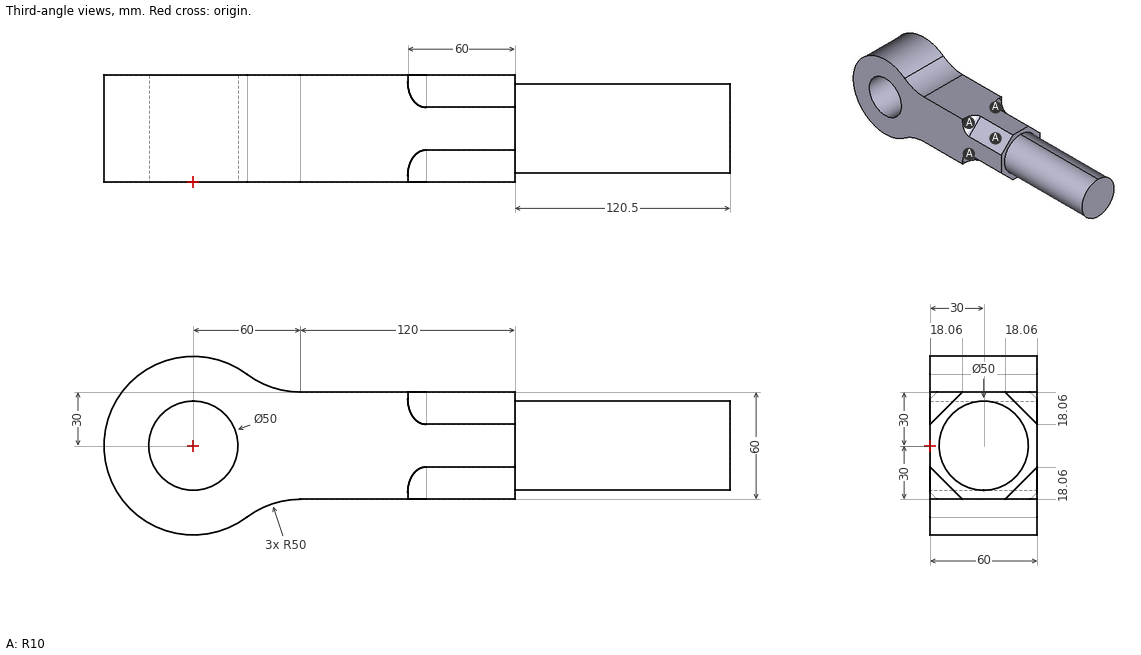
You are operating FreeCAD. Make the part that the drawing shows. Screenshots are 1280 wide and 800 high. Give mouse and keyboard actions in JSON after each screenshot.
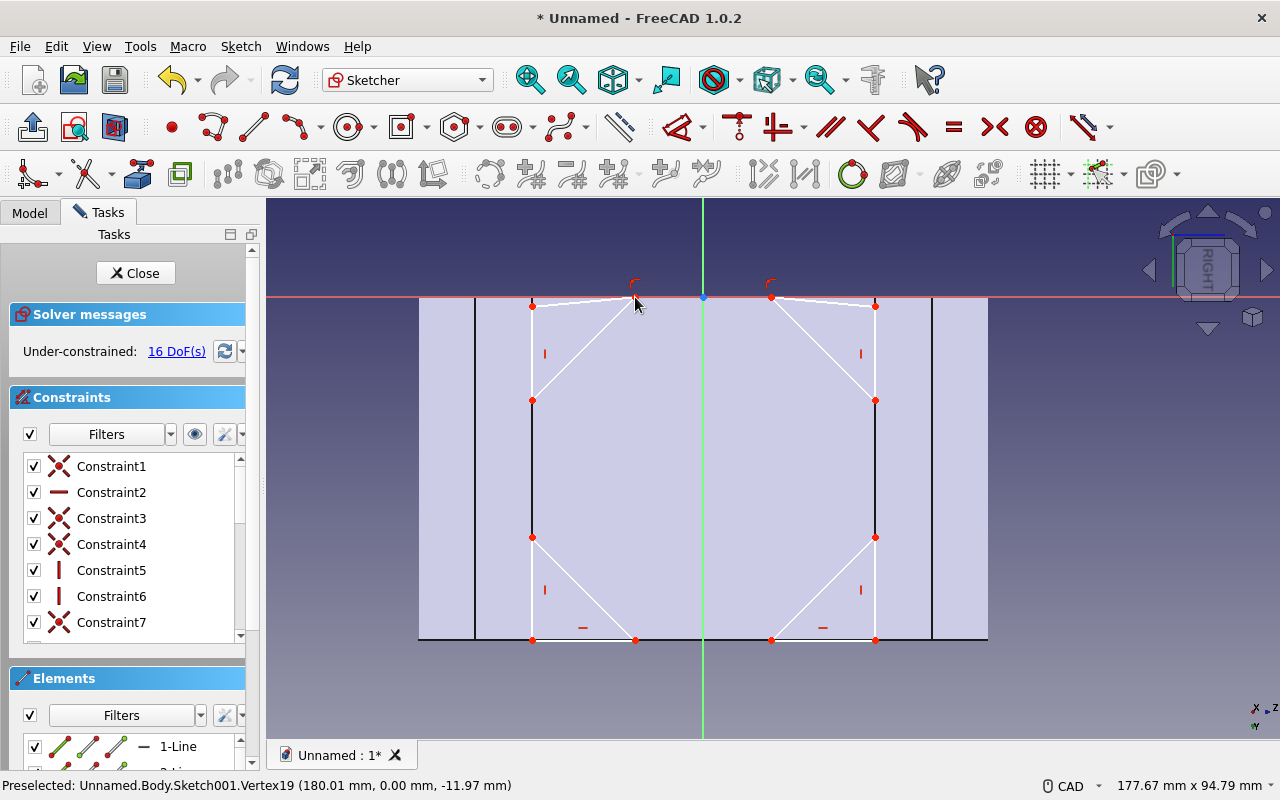
{"action": "left_click", "coordinate": [802, 300]}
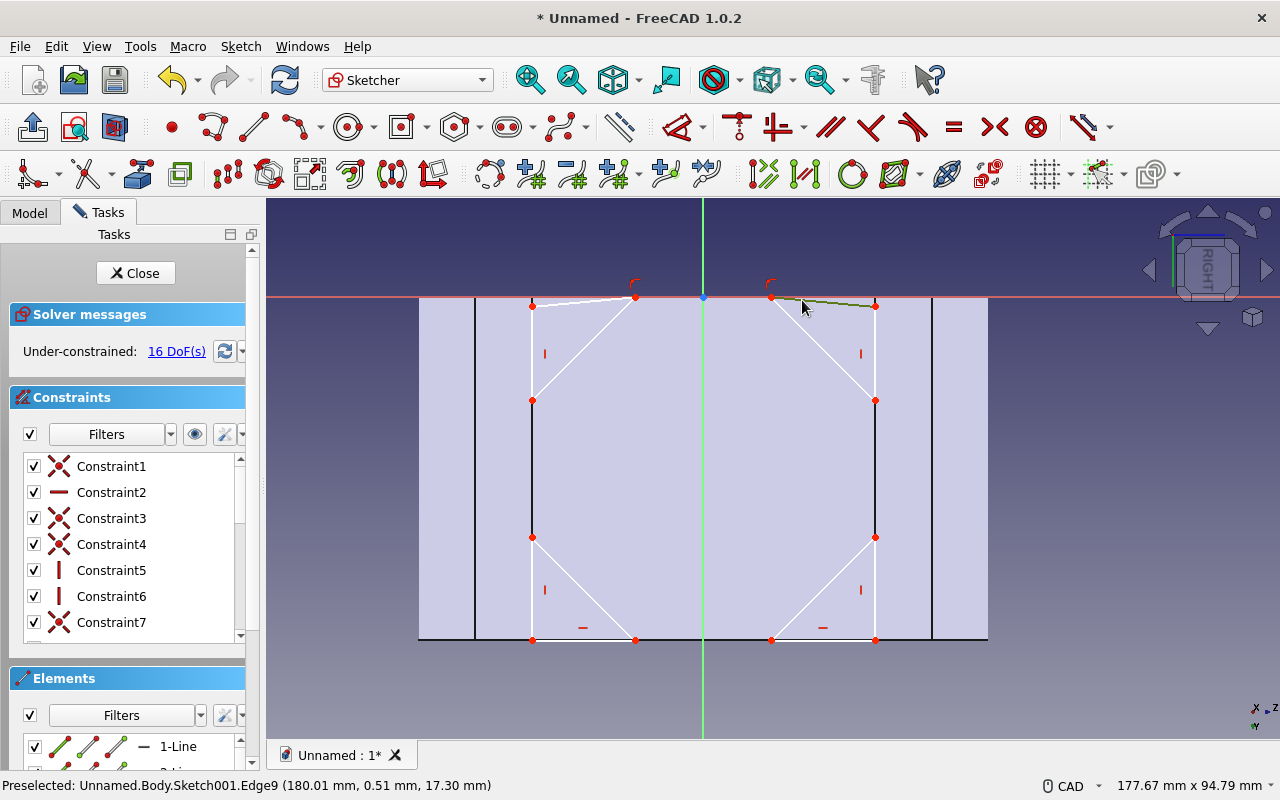
{"action": "key", "text": "h"}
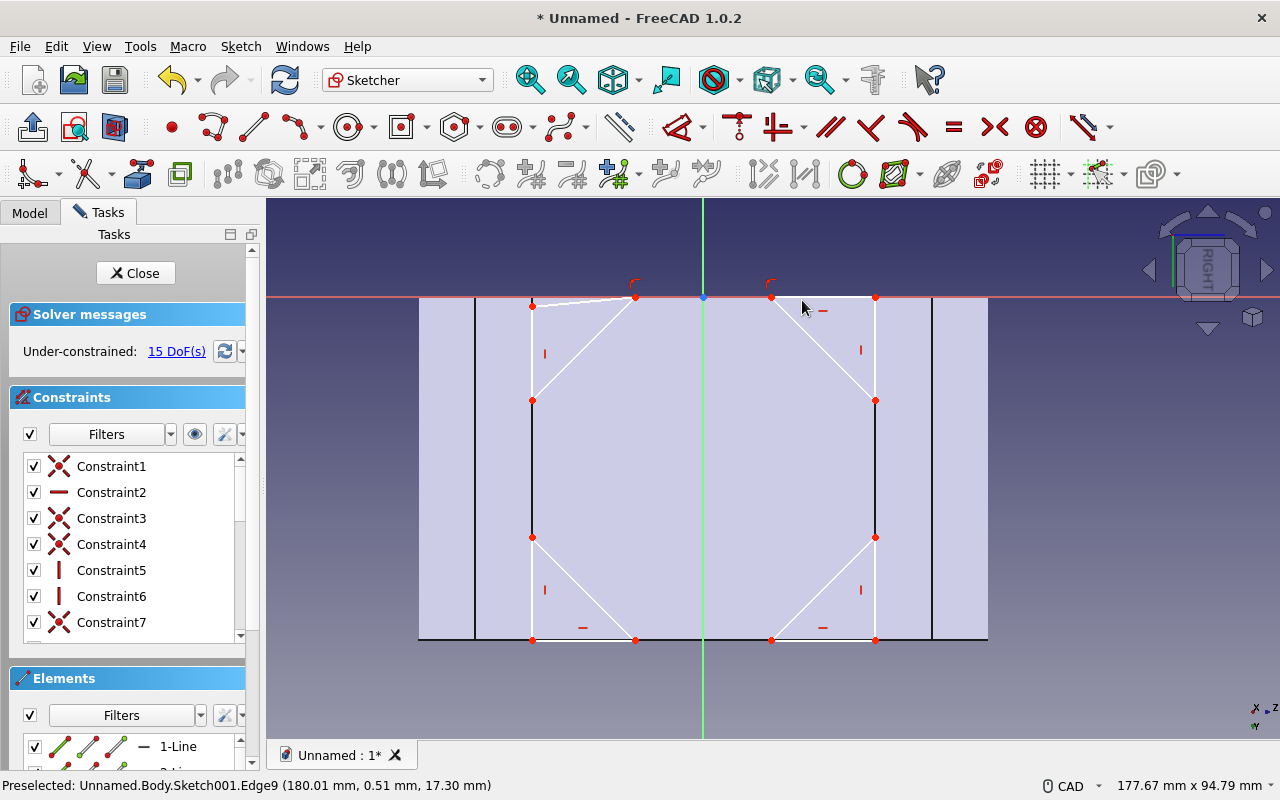
{"action": "left_click", "coordinate": [604, 300]}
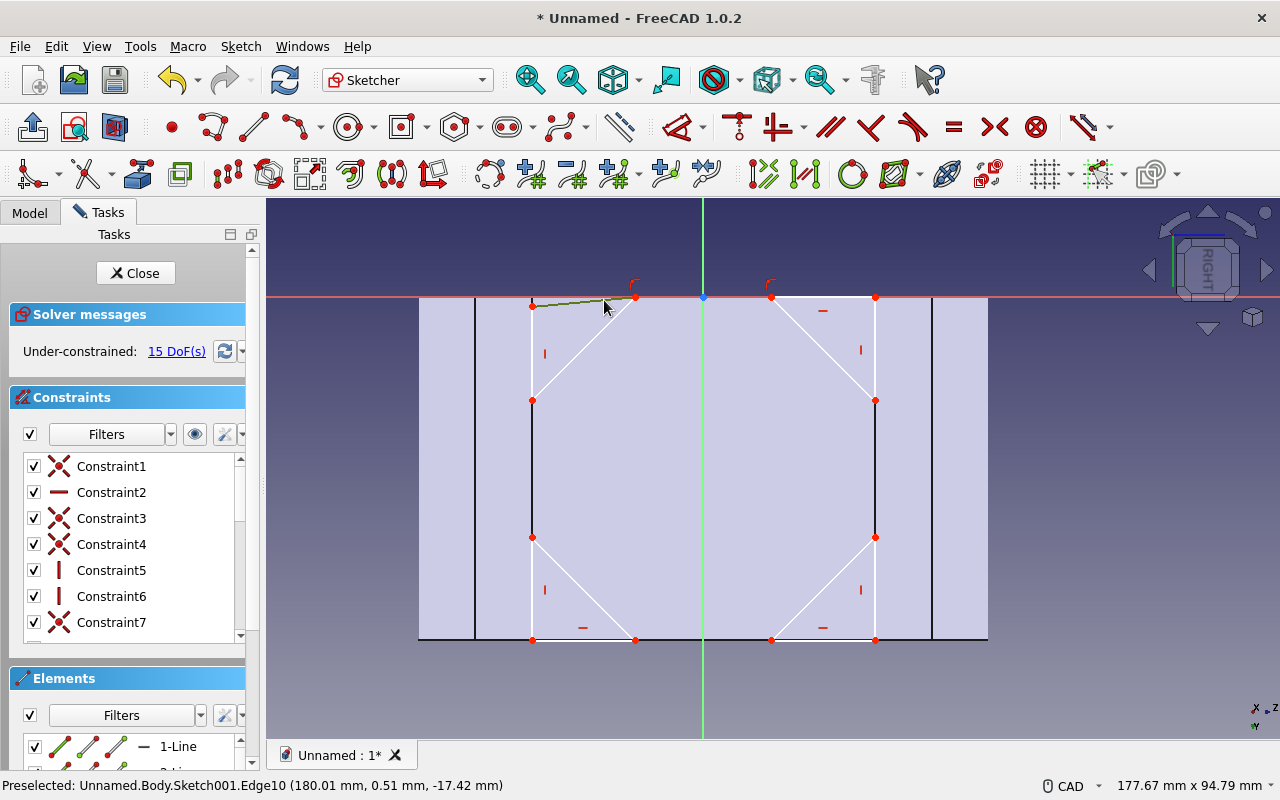
{"action": "key", "text": "h"}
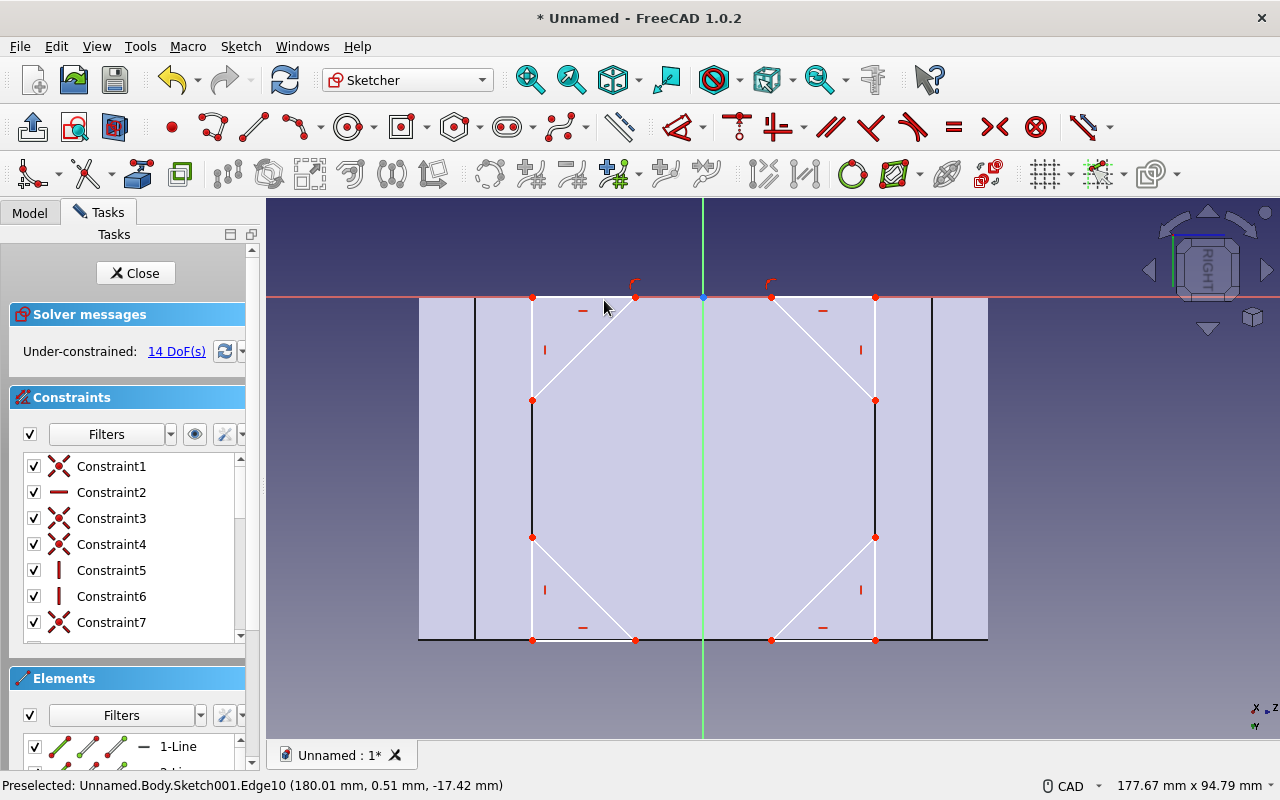
{"action": "key", "text": "d"}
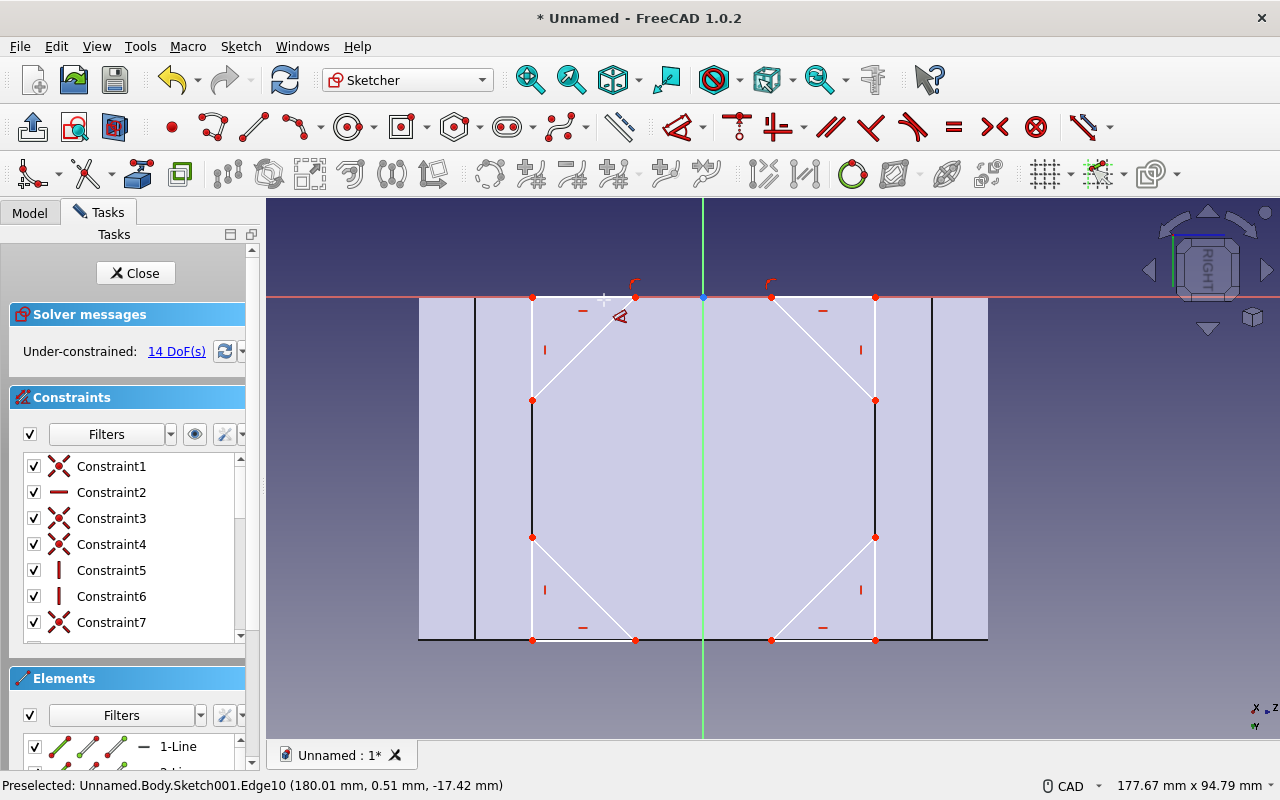
{"action": "left_click", "coordinate": [875, 538]}
{"action": "left_click", "coordinate": [789, 263]}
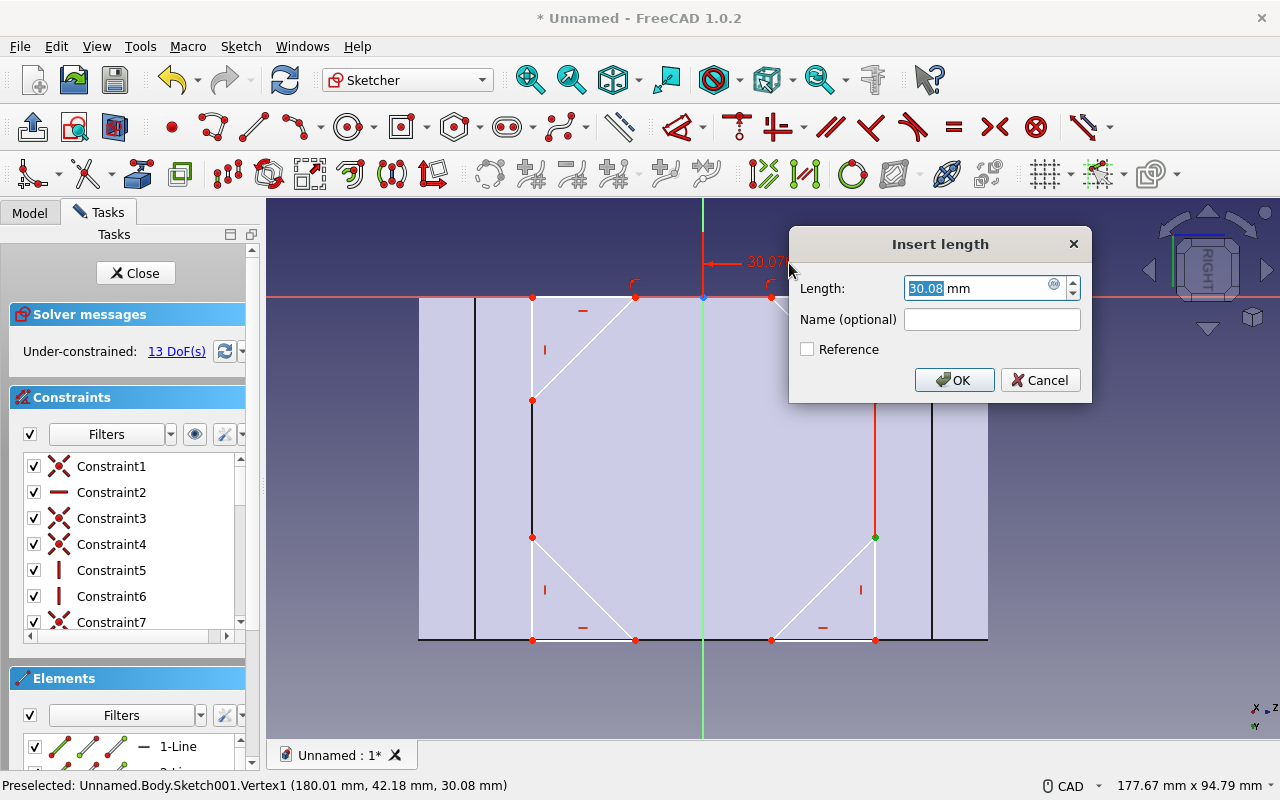
{"action": "type", "text": "30"}
{"action": "key", "text": "Return"}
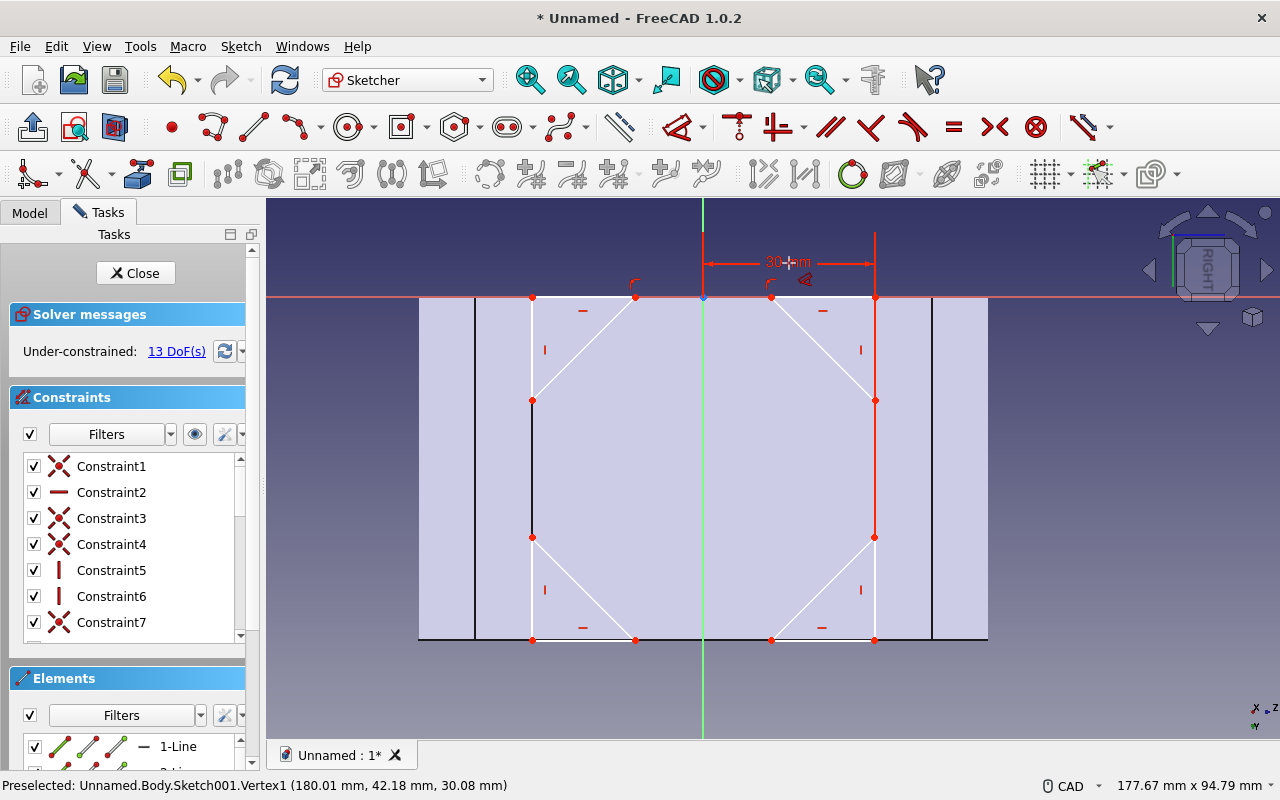
{"action": "left_click", "coordinate": [771, 641]}
{"action": "left_click", "coordinate": [805, 469]}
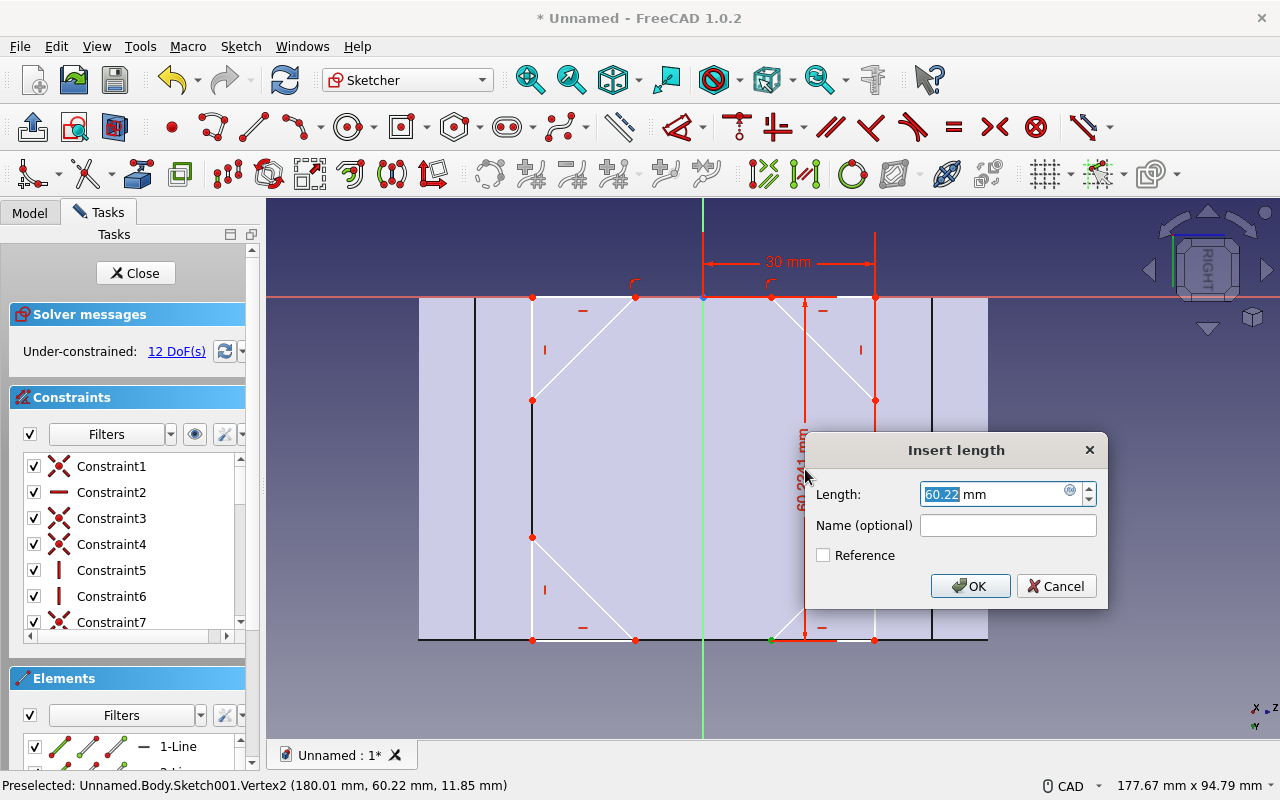
{"action": "type", "text": "60"}
{"action": "key", "text": "Return"}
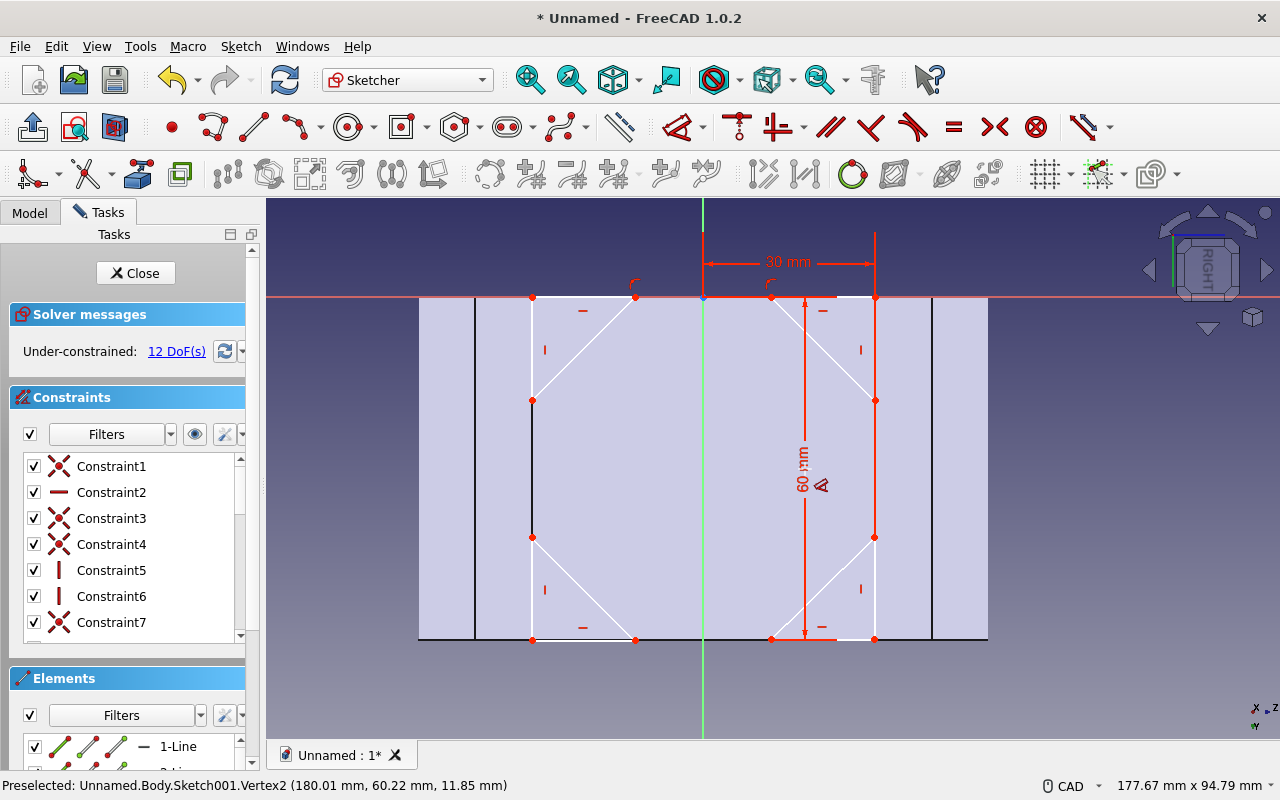
{"action": "left_click", "coordinate": [532, 538]}
{"action": "left_click", "coordinate": [618, 263]}